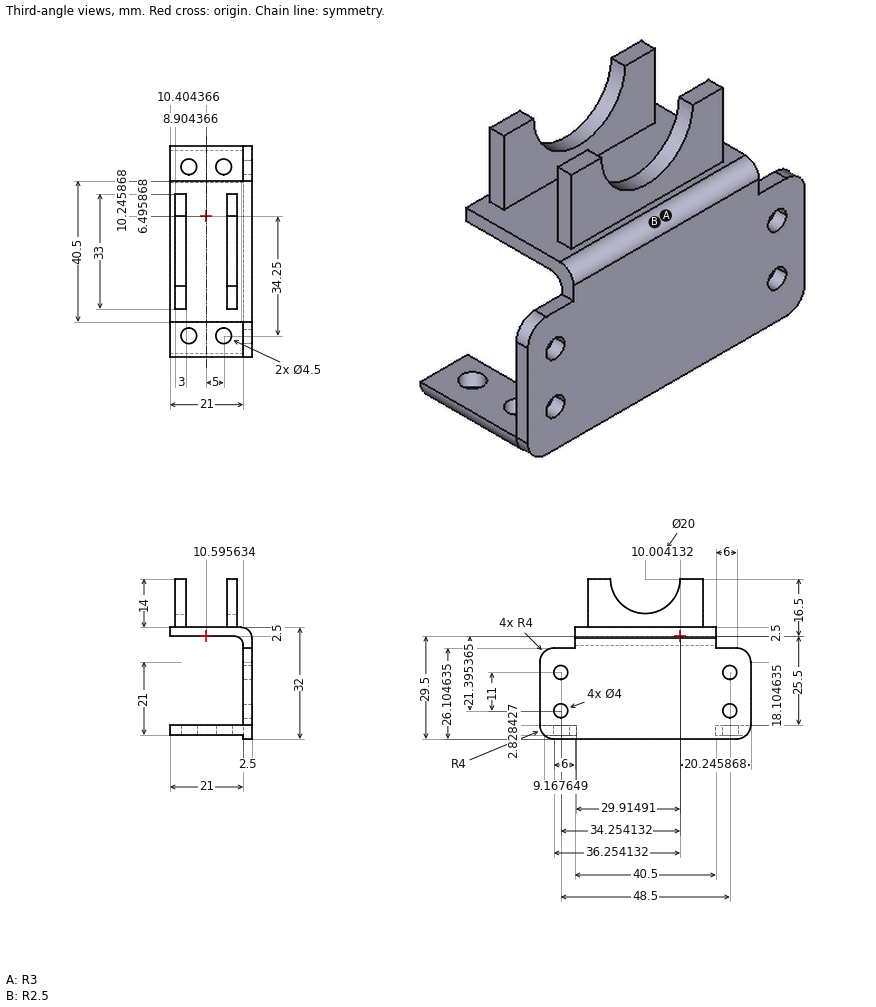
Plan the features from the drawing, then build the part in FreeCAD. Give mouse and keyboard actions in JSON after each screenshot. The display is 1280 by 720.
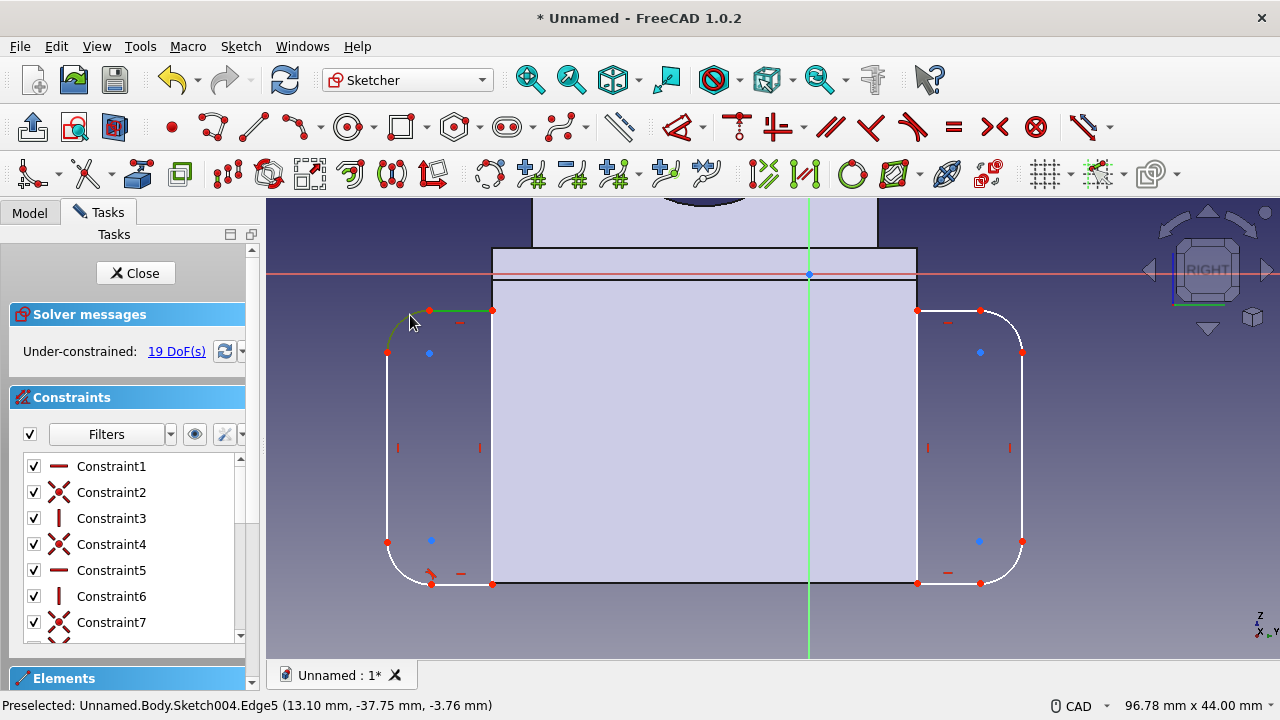
{"action": "left_click", "coordinate": [913, 128]}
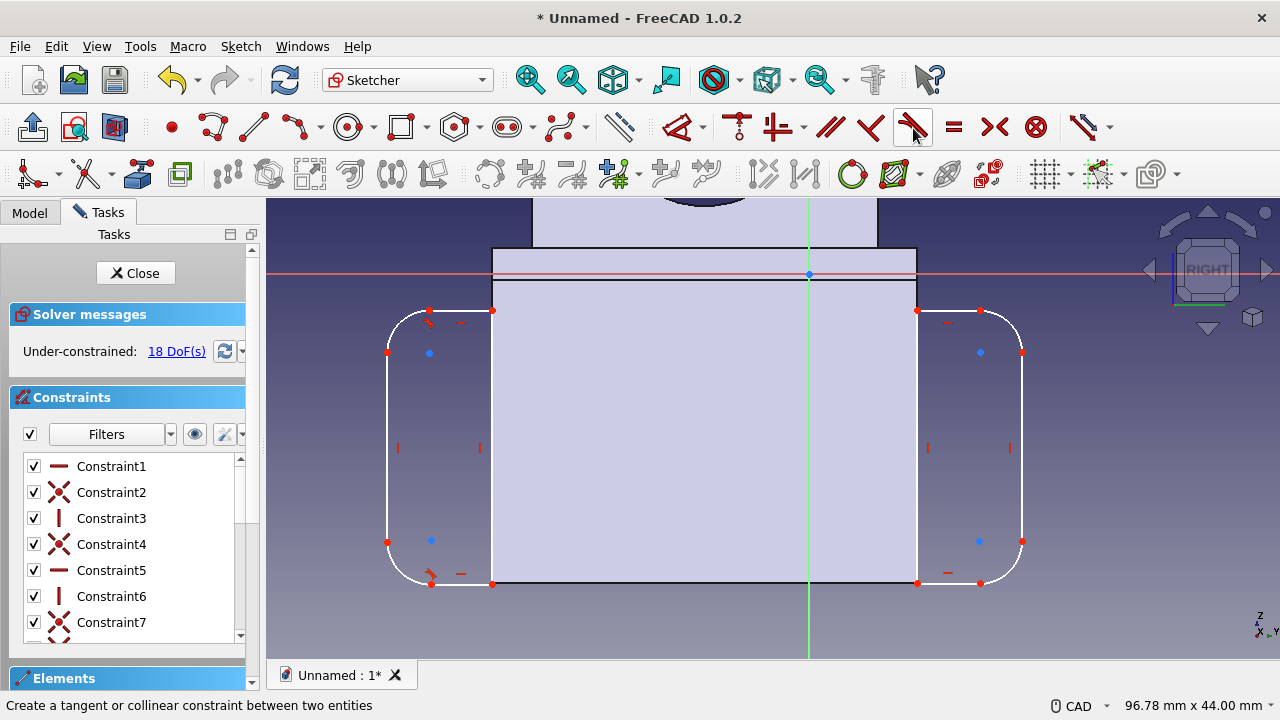
{"action": "left_click", "coordinate": [387, 410]}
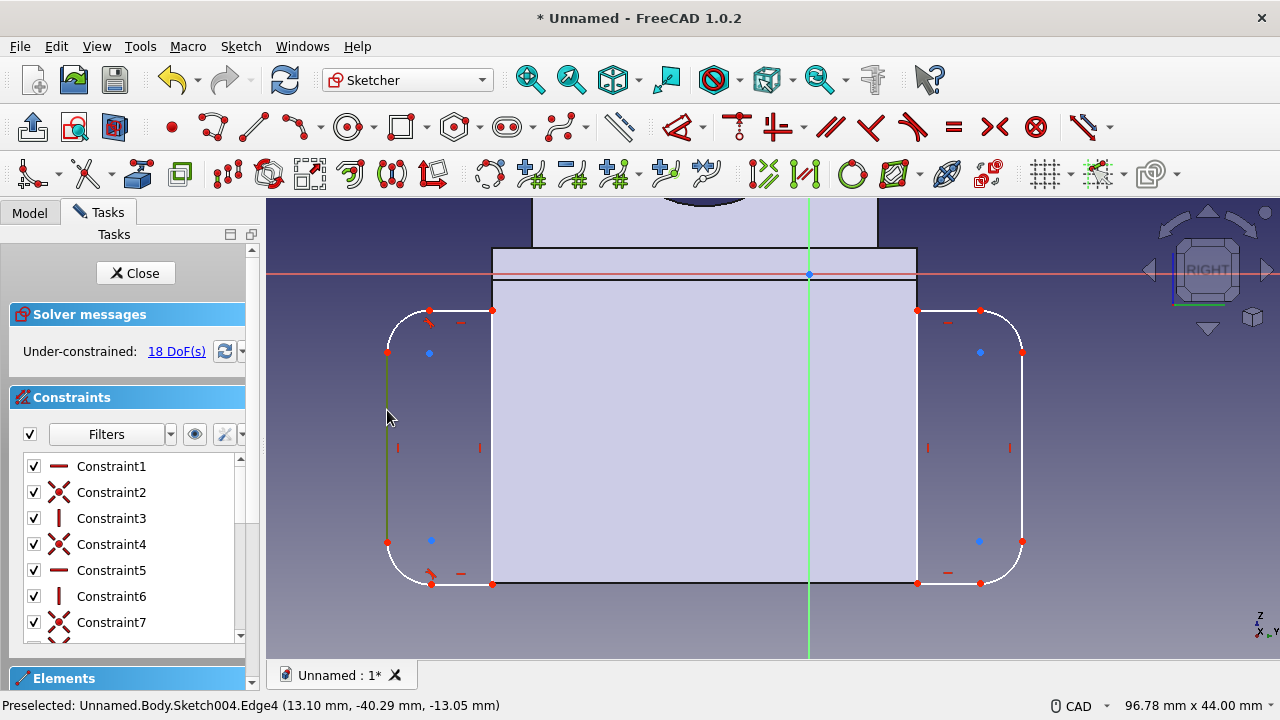
{"action": "left_click", "coordinate": [411, 315]}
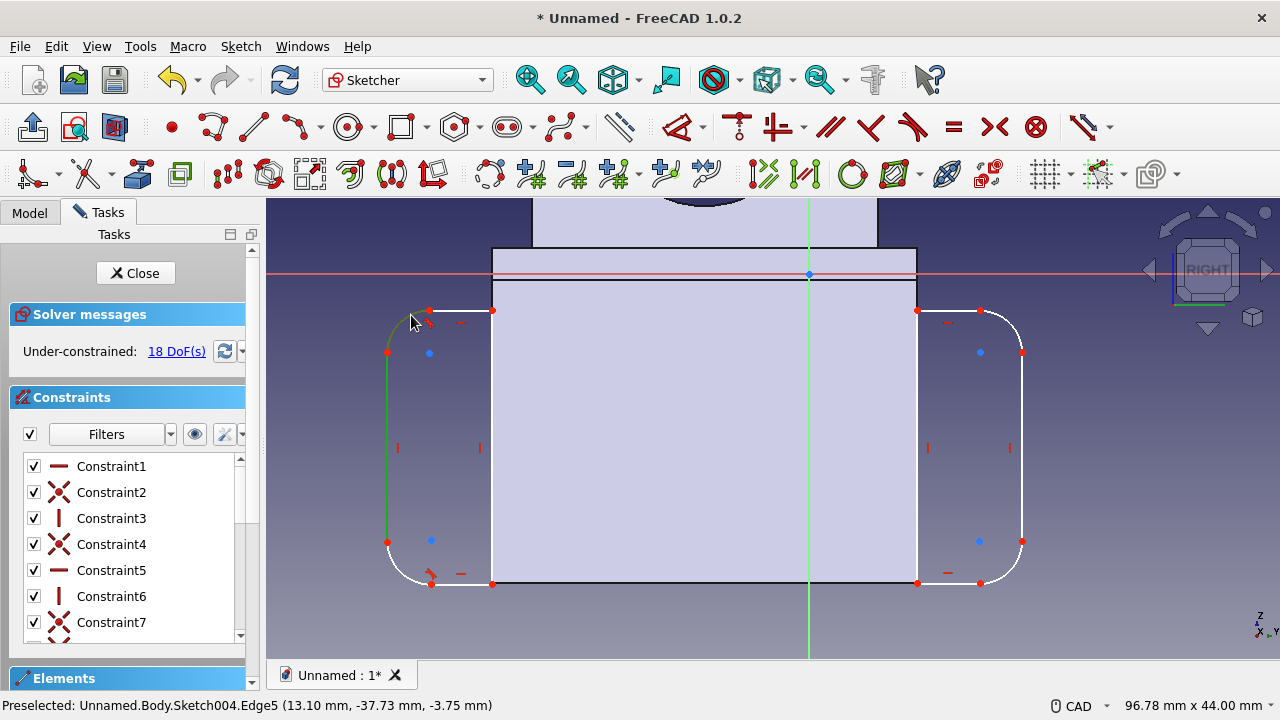
{"action": "left_click", "coordinate": [913, 128]}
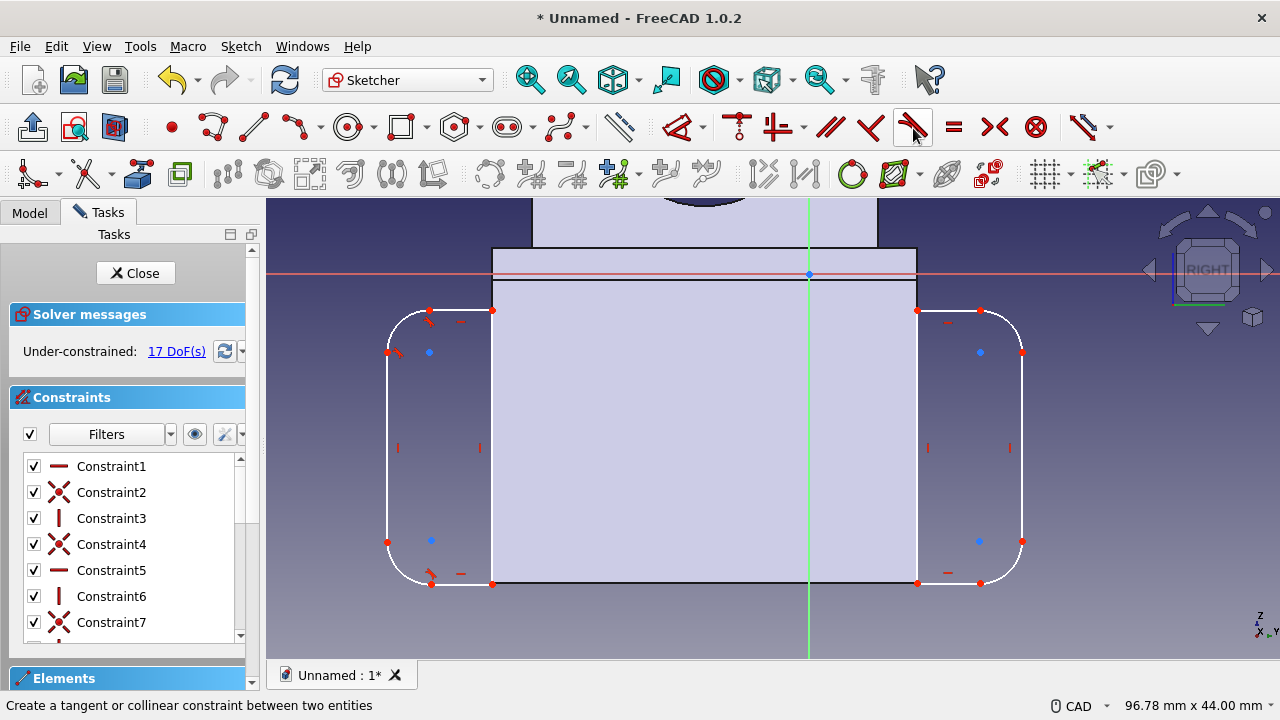
{"action": "left_click", "coordinate": [387, 410]}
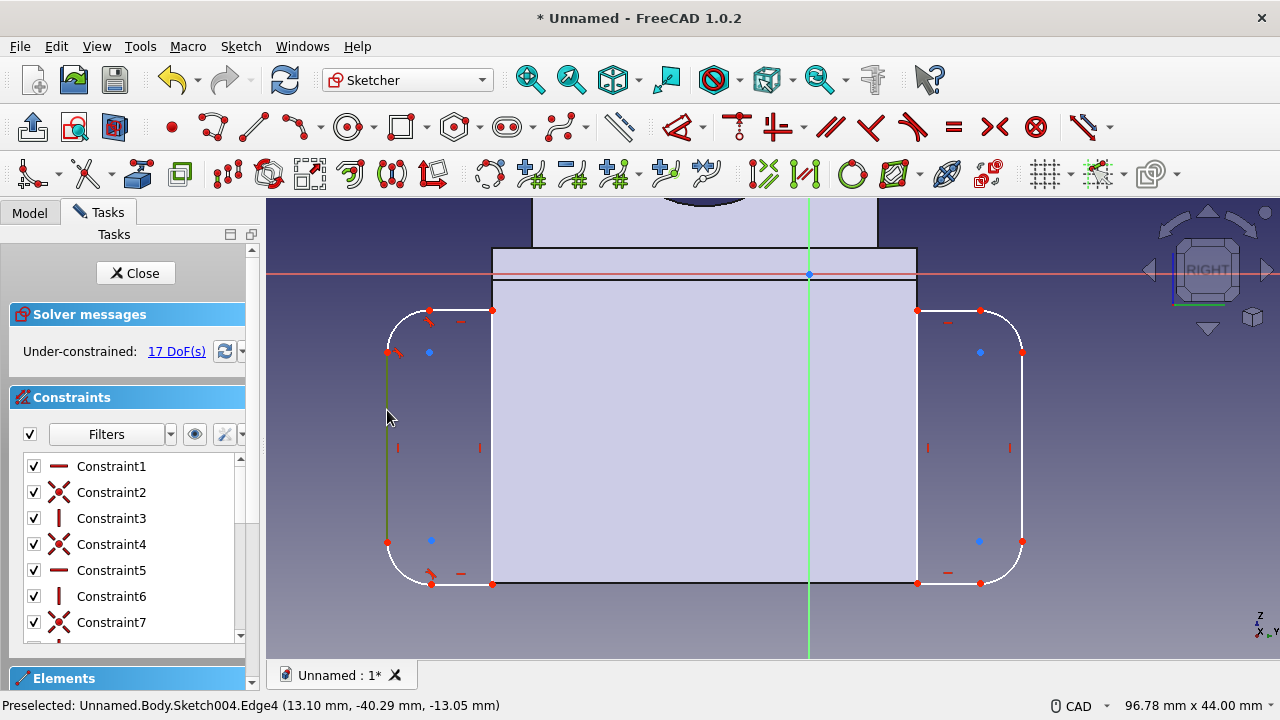
{"action": "left_click", "coordinate": [393, 562]}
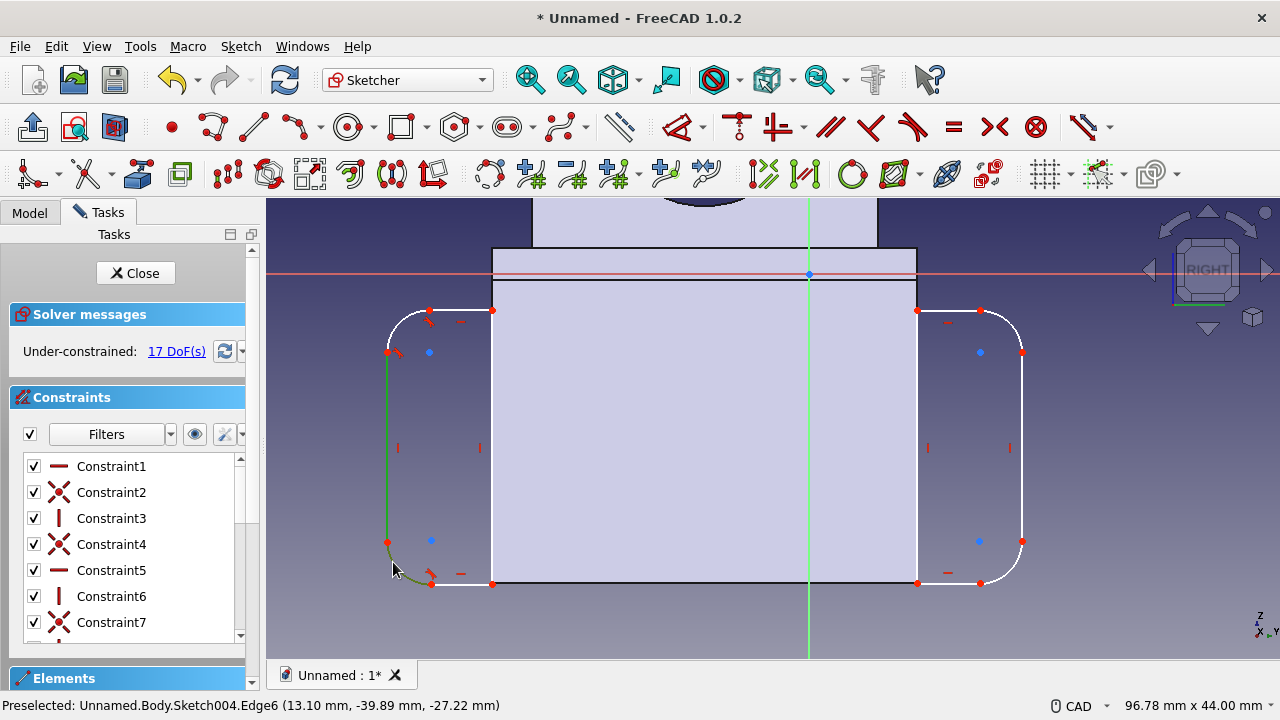
{"action": "left_click", "coordinate": [913, 128]}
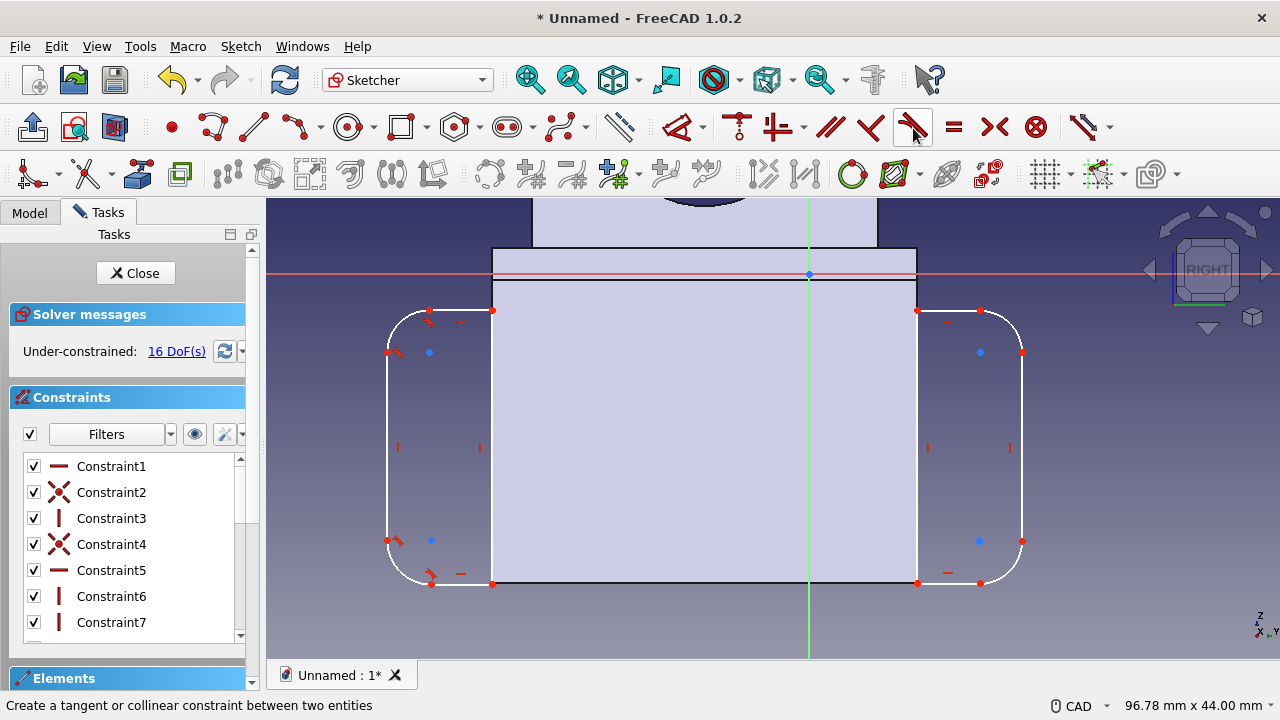
{"action": "left_click", "coordinate": [1022, 485]}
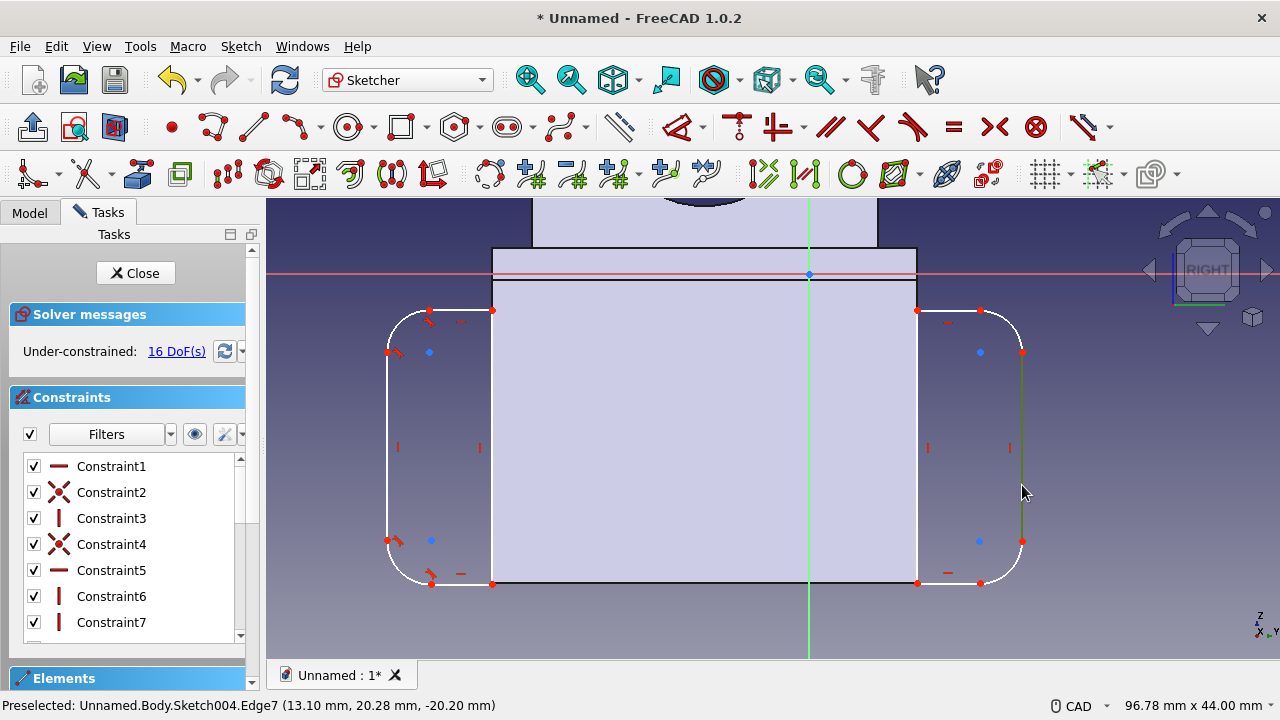
{"action": "left_click", "coordinate": [1017, 334]}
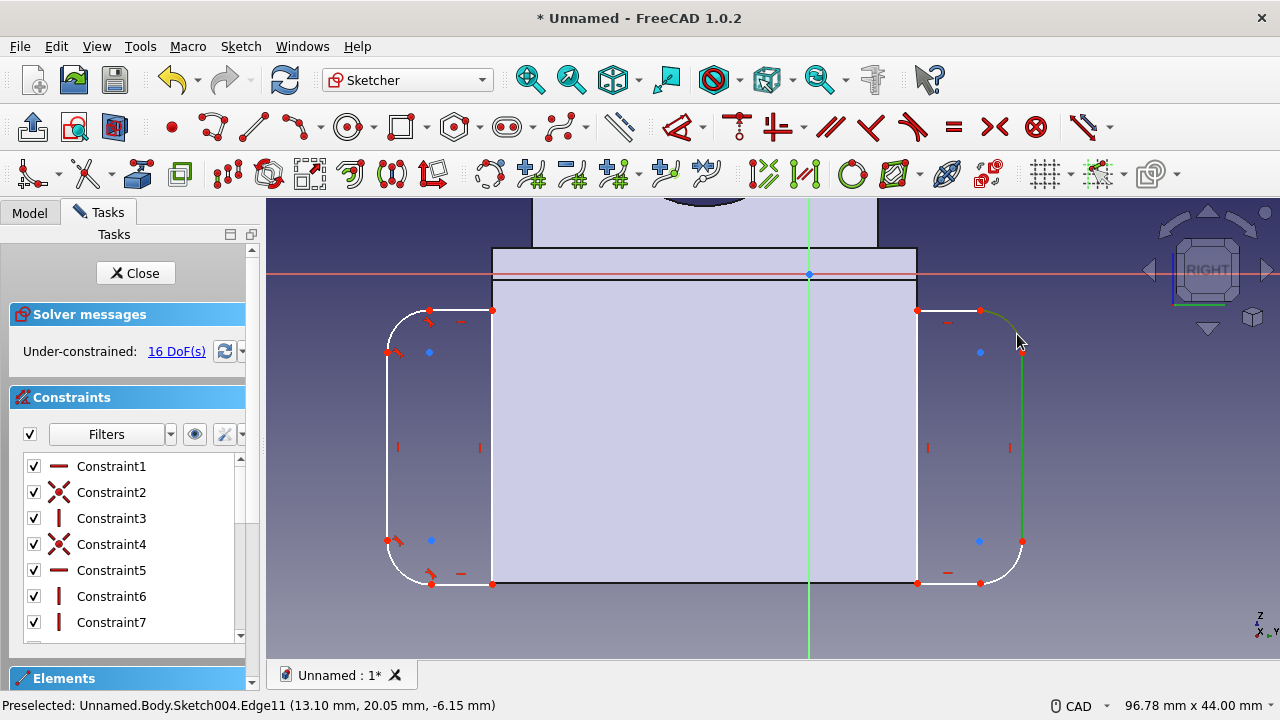
{"action": "key", "text": "t"}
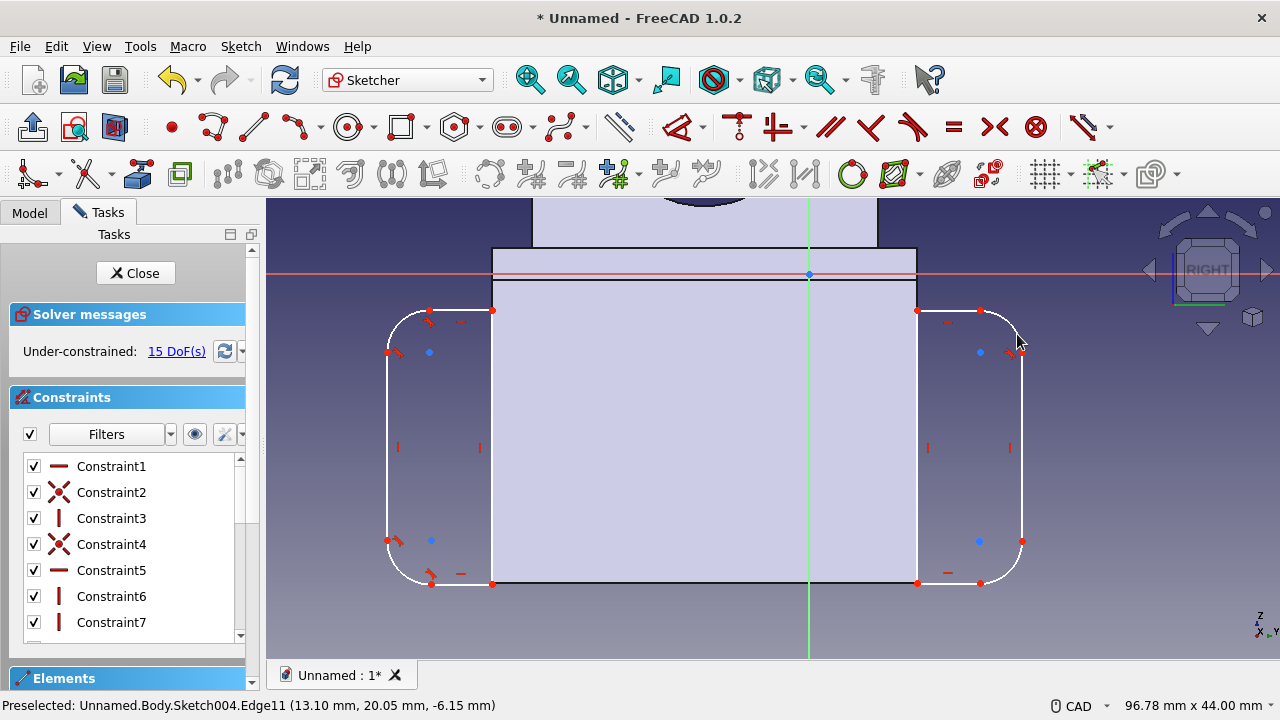
{"action": "left_click", "coordinate": [1022, 485]}